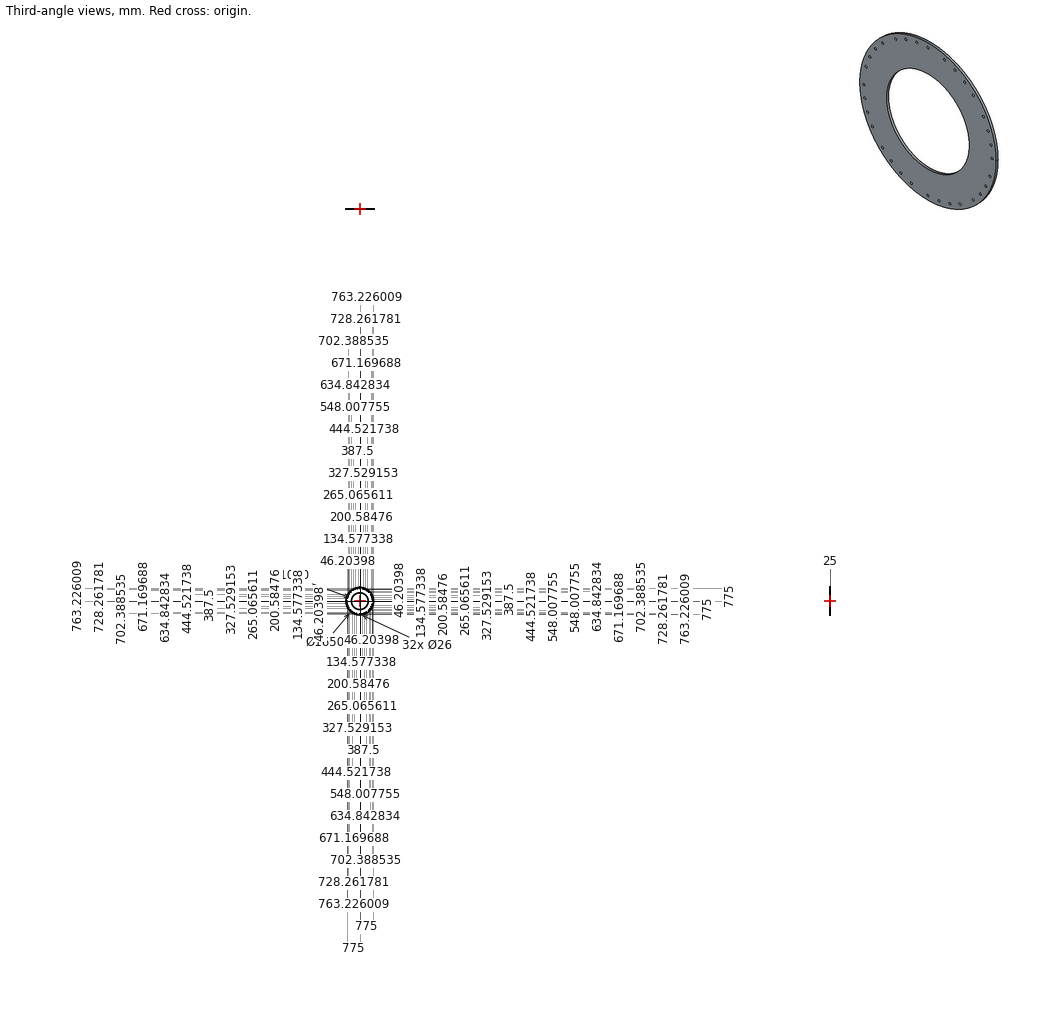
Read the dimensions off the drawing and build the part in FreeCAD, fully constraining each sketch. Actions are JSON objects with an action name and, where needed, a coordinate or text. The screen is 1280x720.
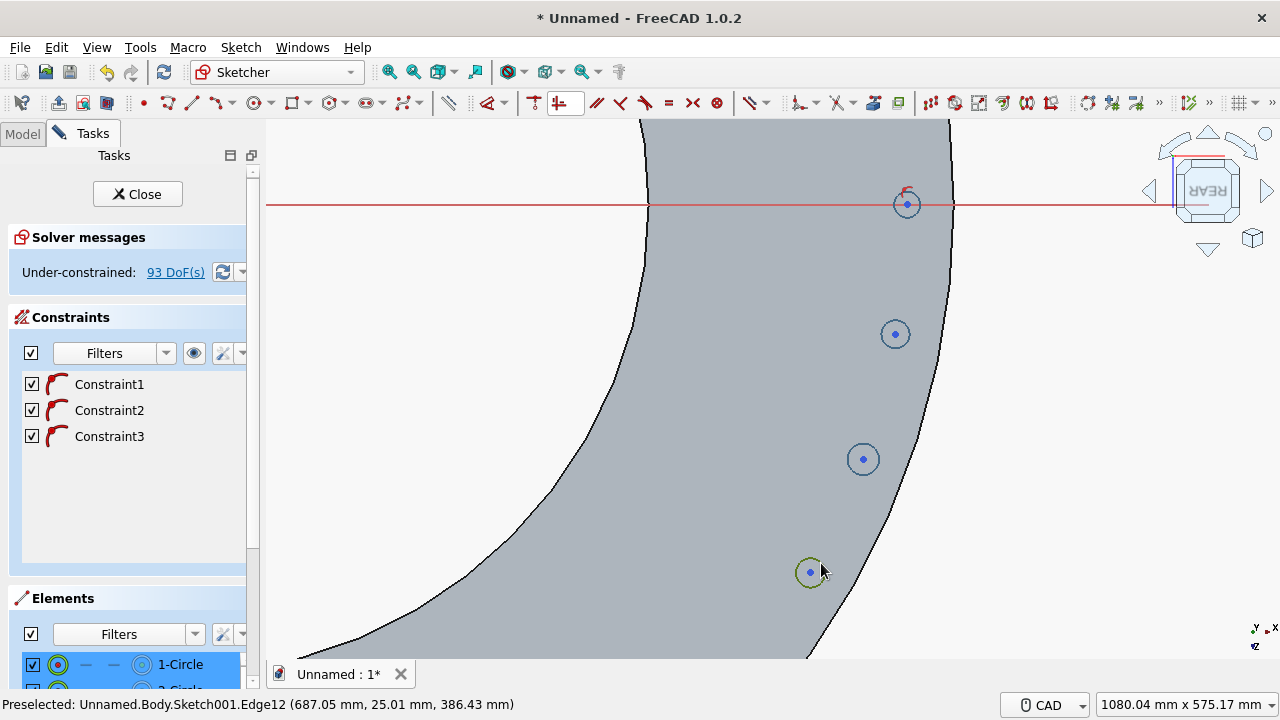
{"action": "scroll", "coordinate": [876, 449], "scroll_direction": "down", "scroll_amount": 7}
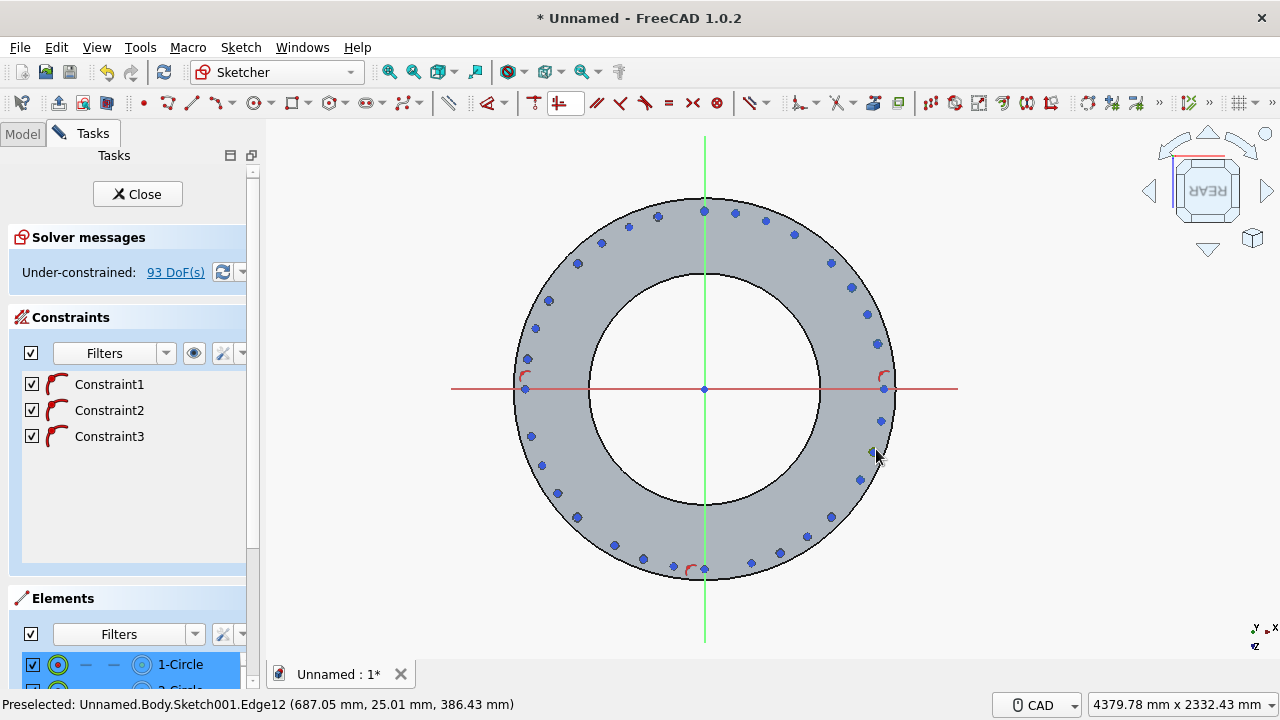
{"action": "scroll", "coordinate": [834, 514], "scroll_direction": "up", "scroll_amount": 7}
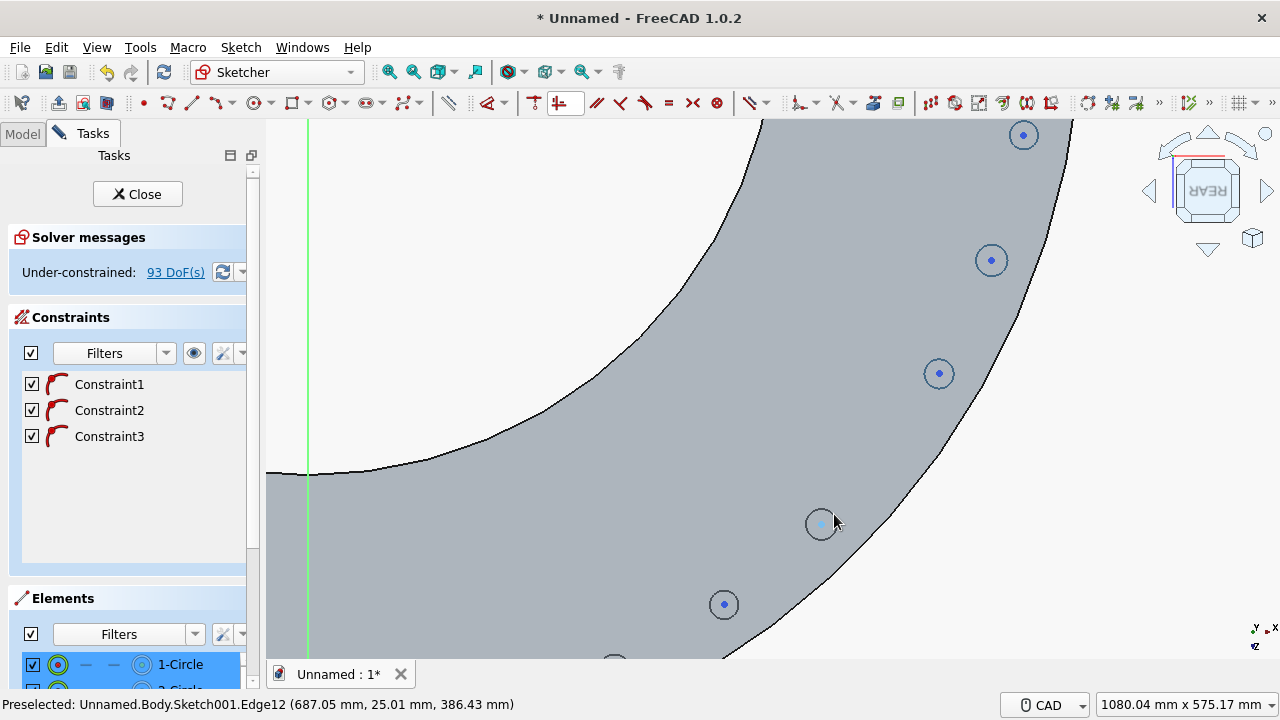
{"action": "left_click", "coordinate": [832, 513]}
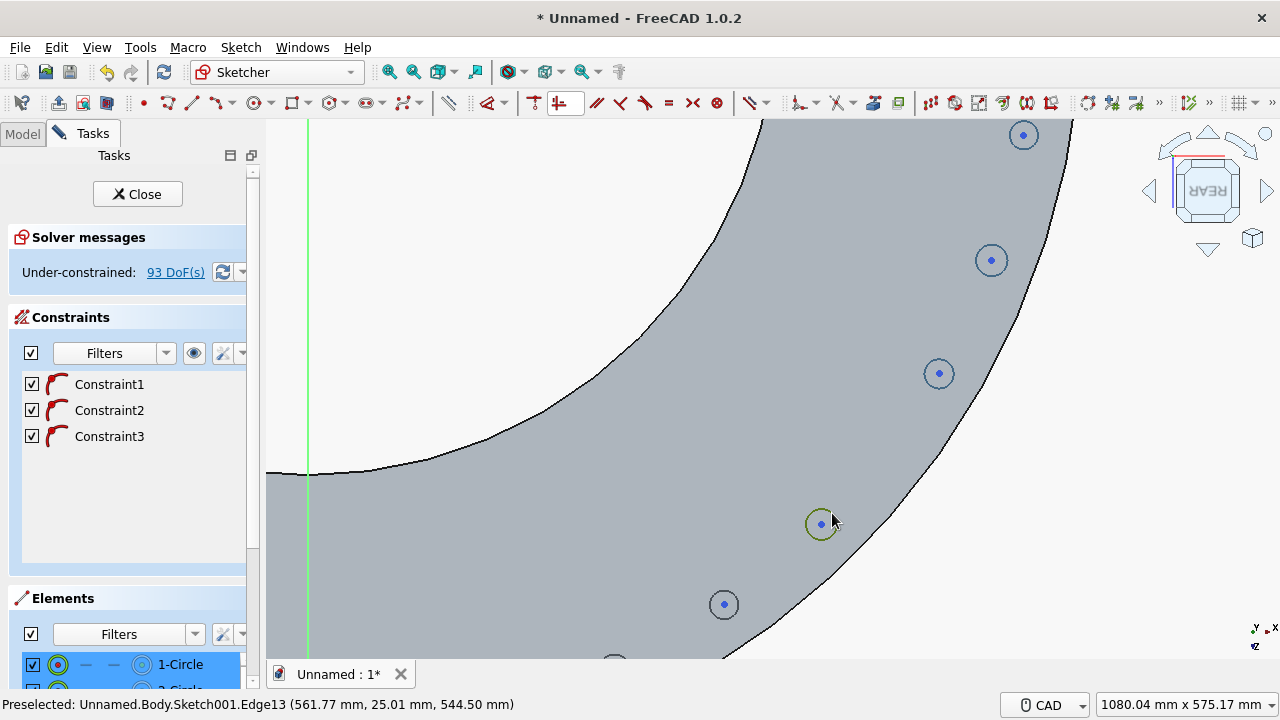
{"action": "left_click", "coordinate": [734, 595]}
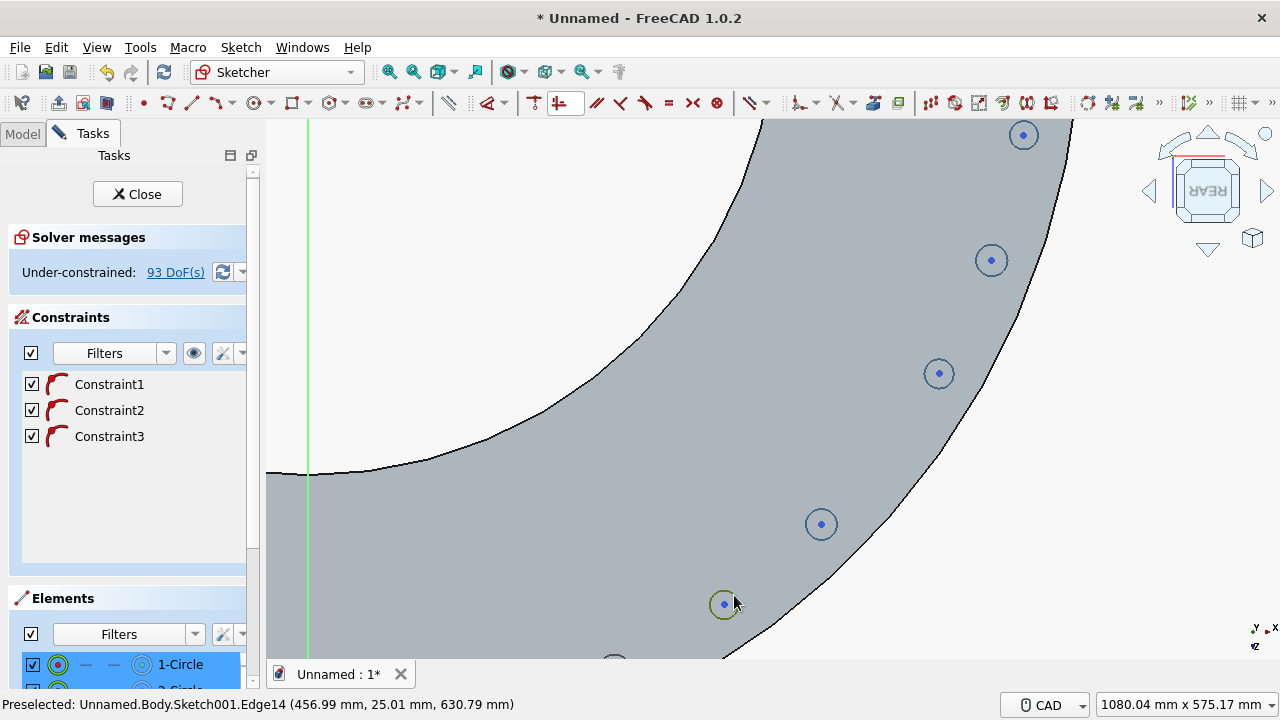
{"action": "scroll", "coordinate": [834, 514], "scroll_direction": "down", "scroll_amount": 7}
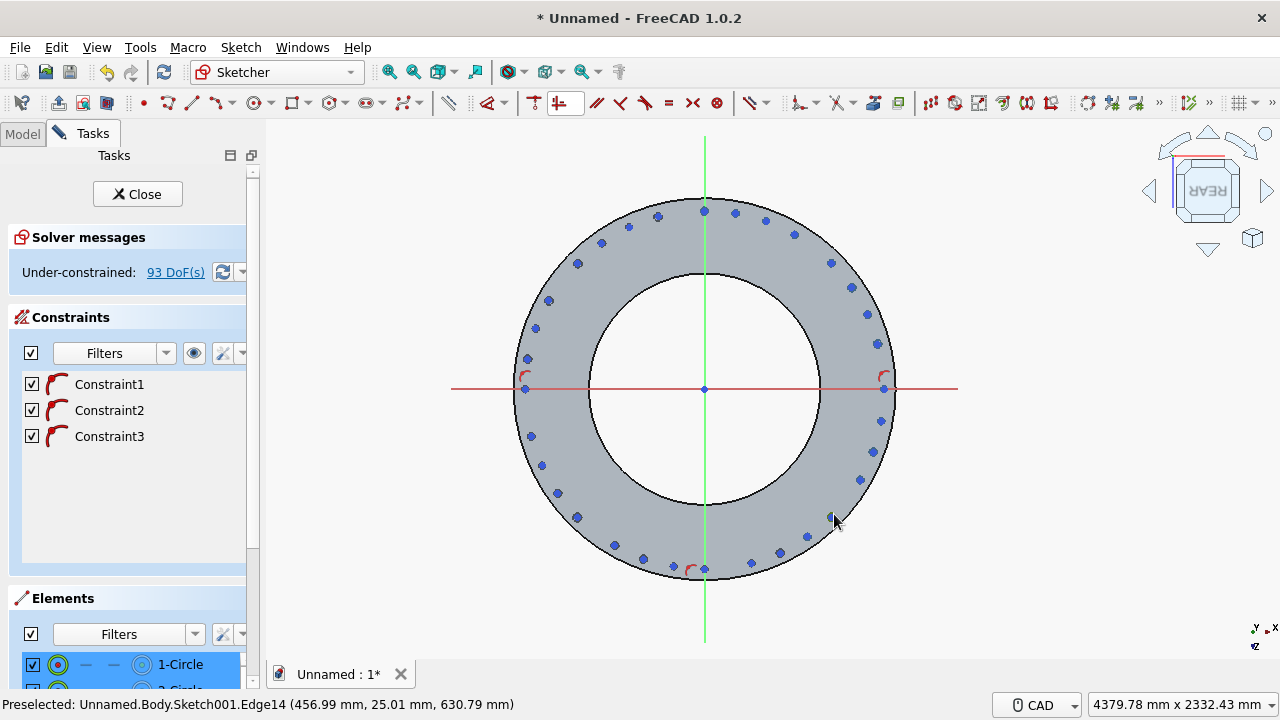
{"action": "scroll", "coordinate": [783, 550], "scroll_direction": "up", "scroll_amount": 7}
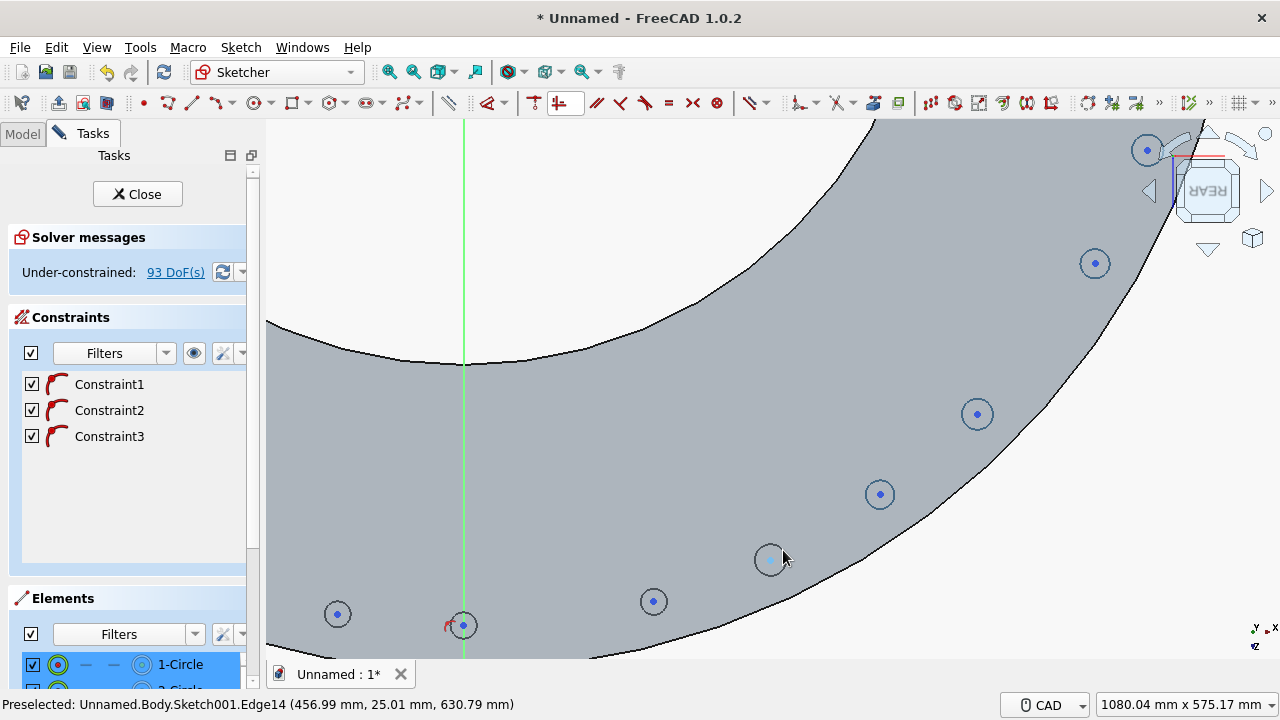
{"action": "left_click", "coordinate": [782, 549]}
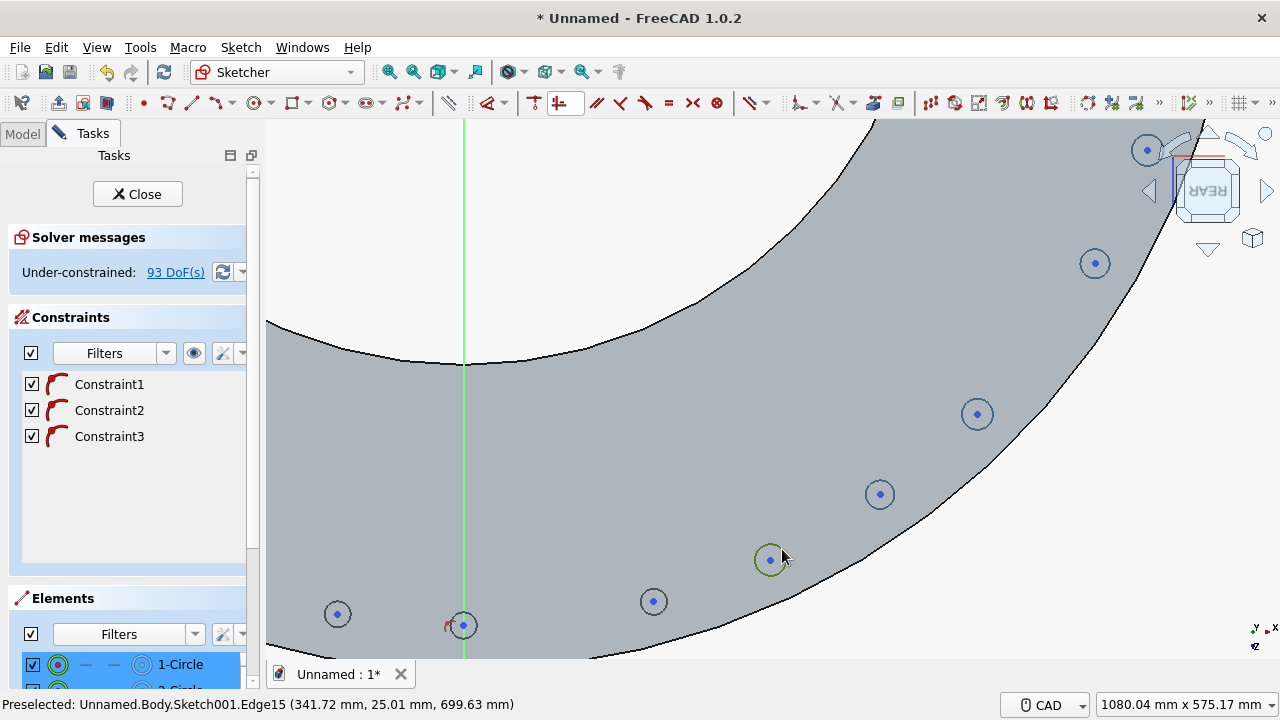
{"action": "left_click", "coordinate": [663, 593]}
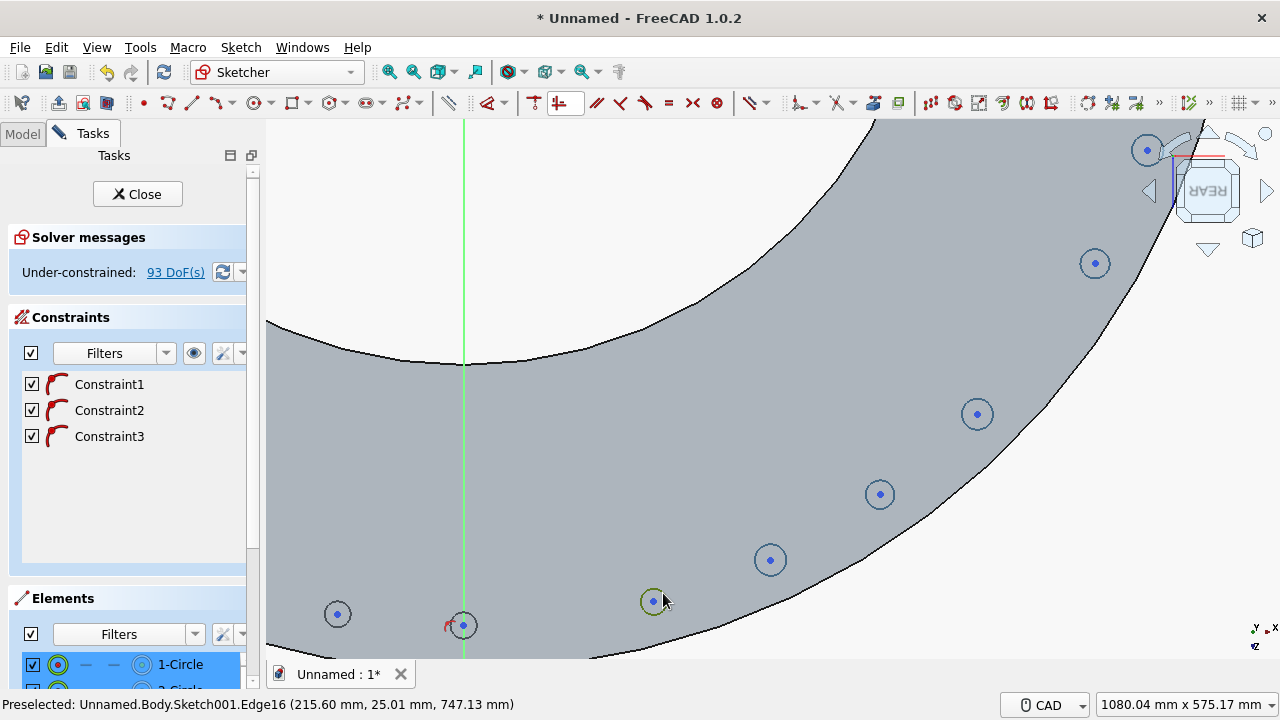
{"action": "scroll", "coordinate": [473, 616], "scroll_direction": "up", "scroll_amount": 3}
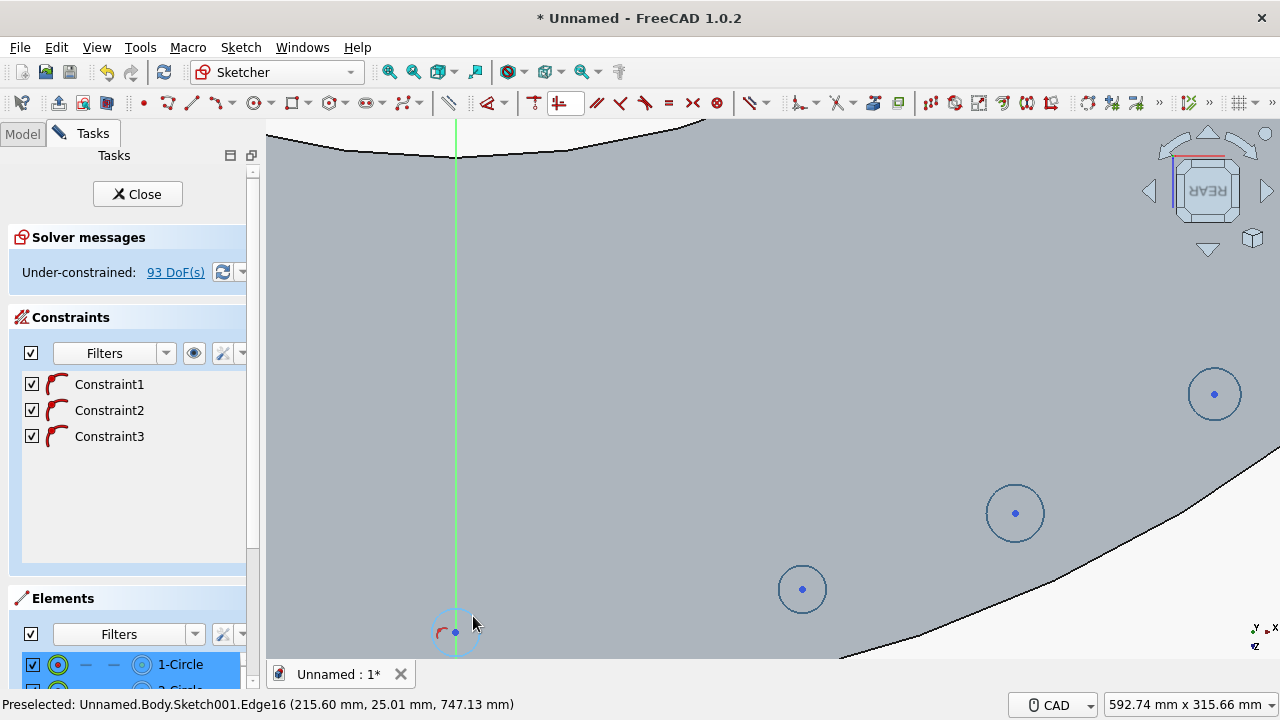
{"action": "left_click", "coordinate": [473, 616]}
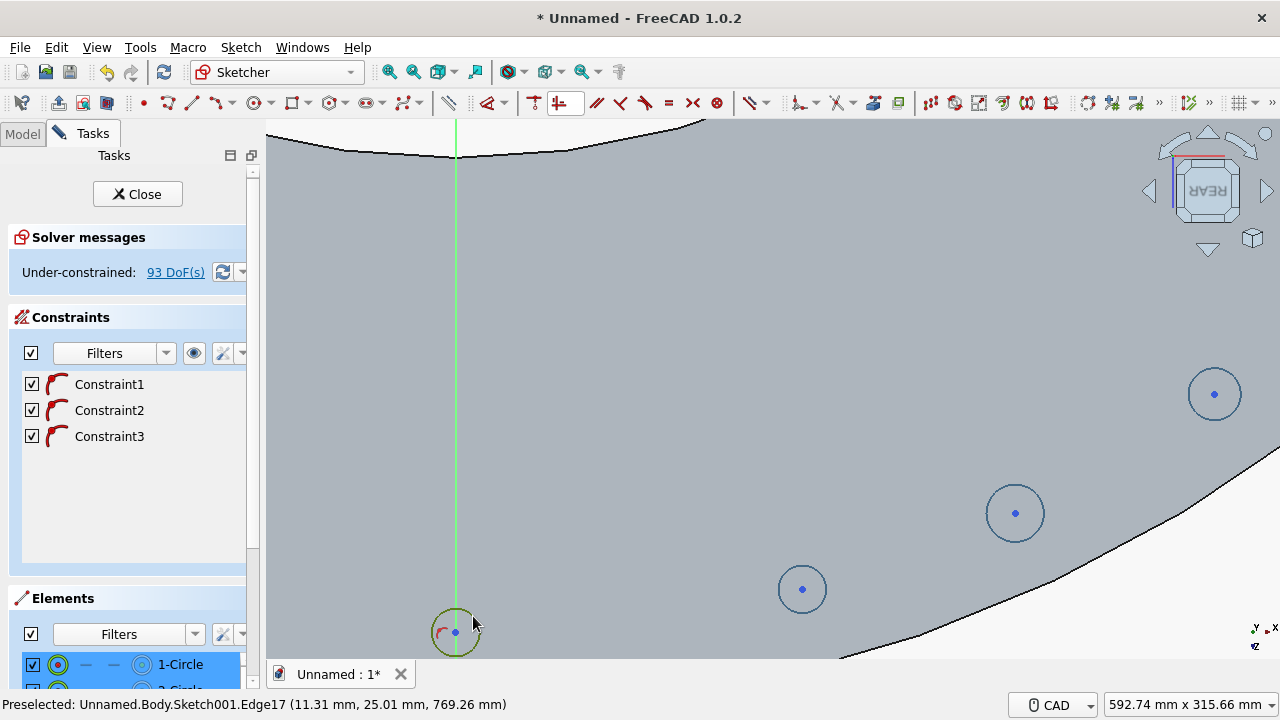
{"action": "scroll", "coordinate": [743, 559], "scroll_direction": "down", "scroll_amount": 10}